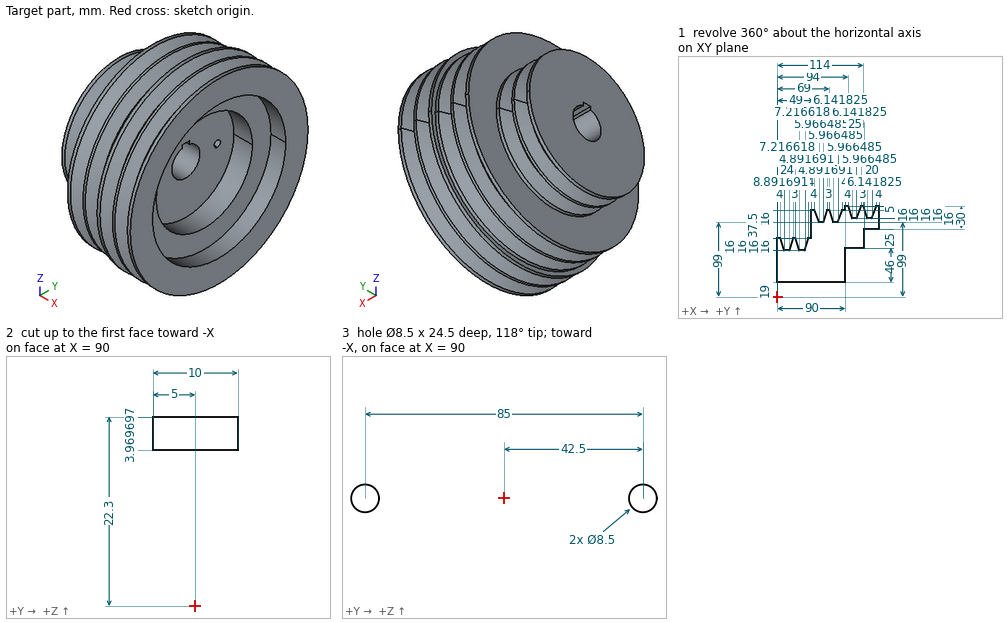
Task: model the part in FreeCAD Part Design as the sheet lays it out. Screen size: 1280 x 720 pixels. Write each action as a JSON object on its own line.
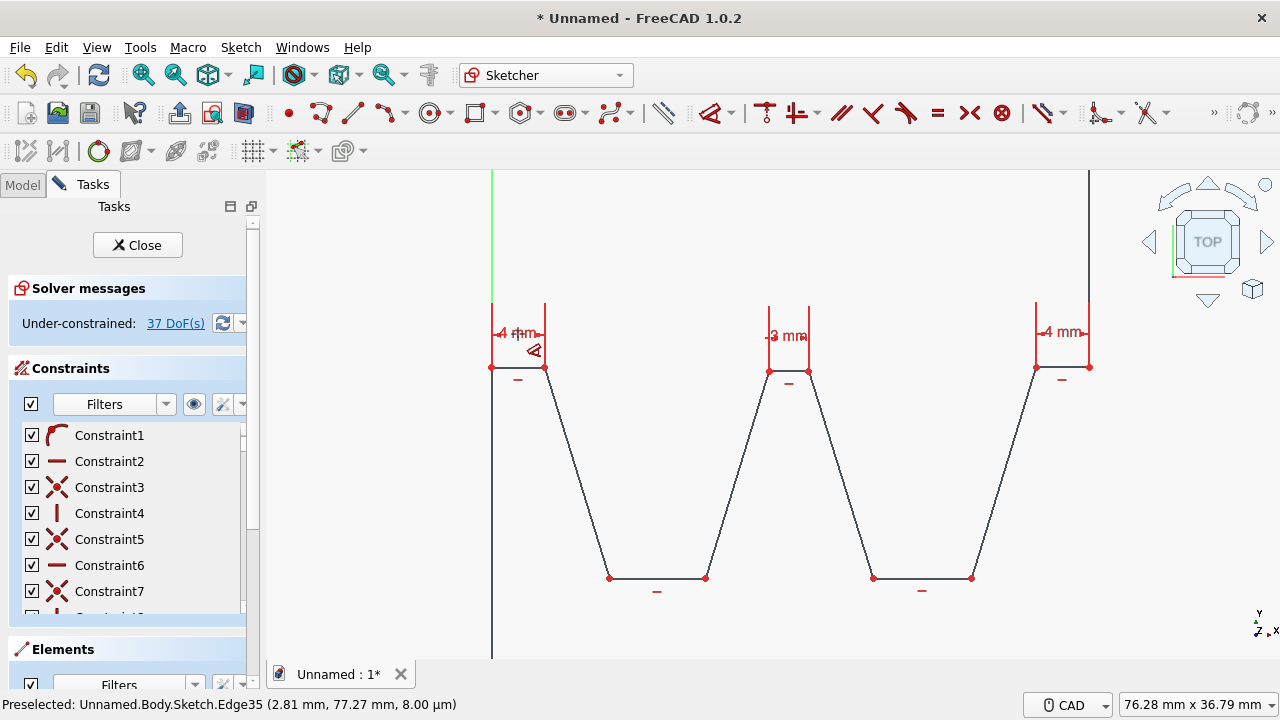
{"action": "scroll", "coordinate": [531, 368], "scroll_direction": "down", "scroll_amount": 8}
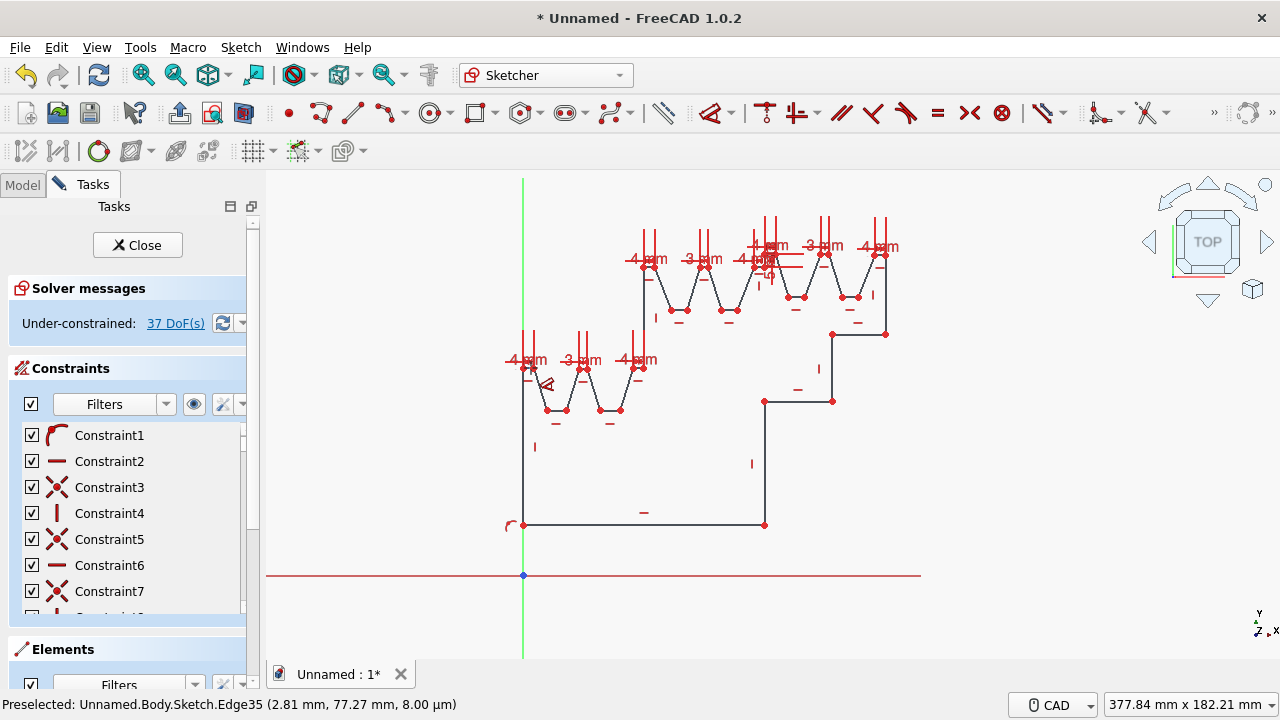
{"action": "left_click", "coordinate": [596, 525]}
{"action": "left_click", "coordinate": [644, 559]}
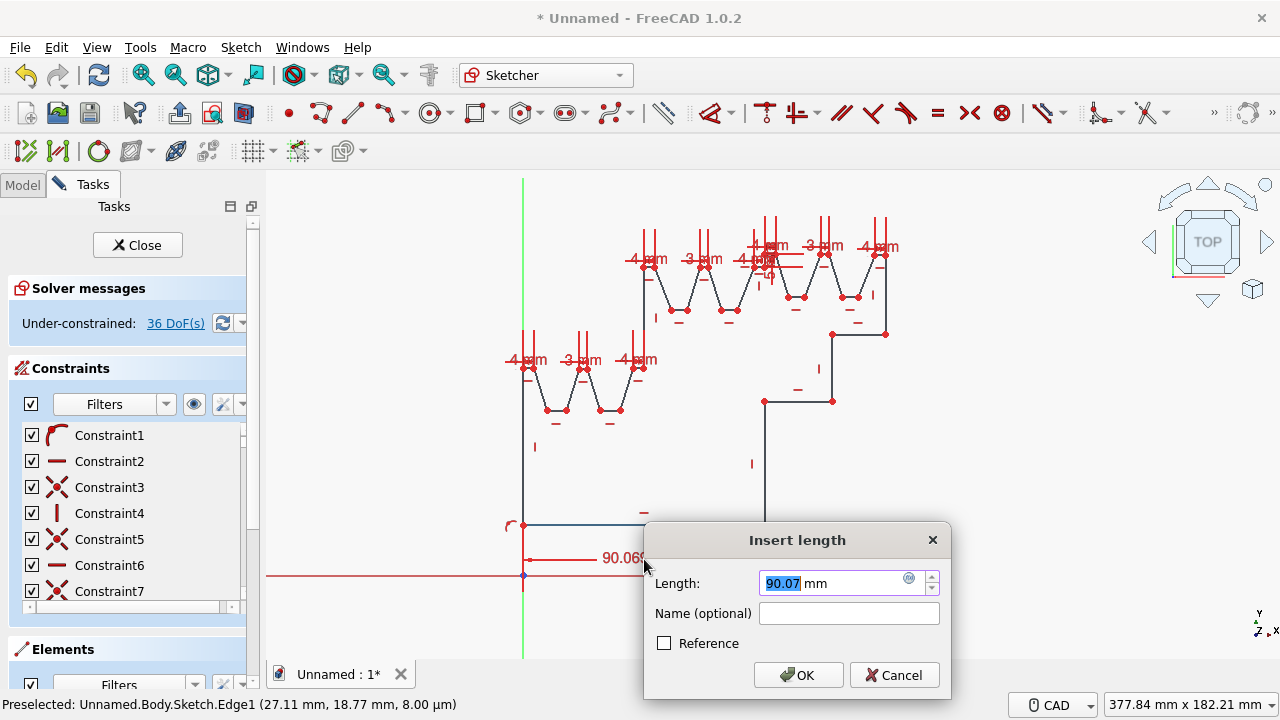
{"action": "type", "text": "90"}
{"action": "key", "text": "Return"}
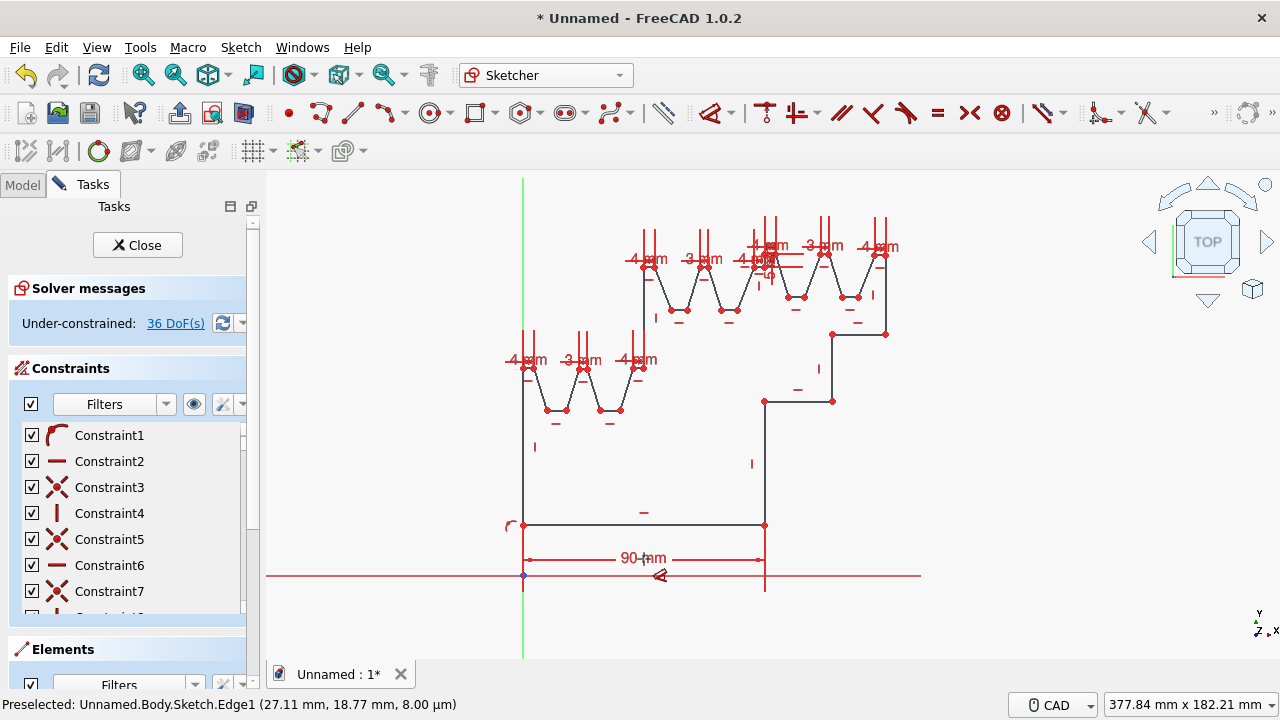
{"action": "left_click", "coordinate": [765, 488]}
{"action": "left_click", "coordinate": [799, 464]}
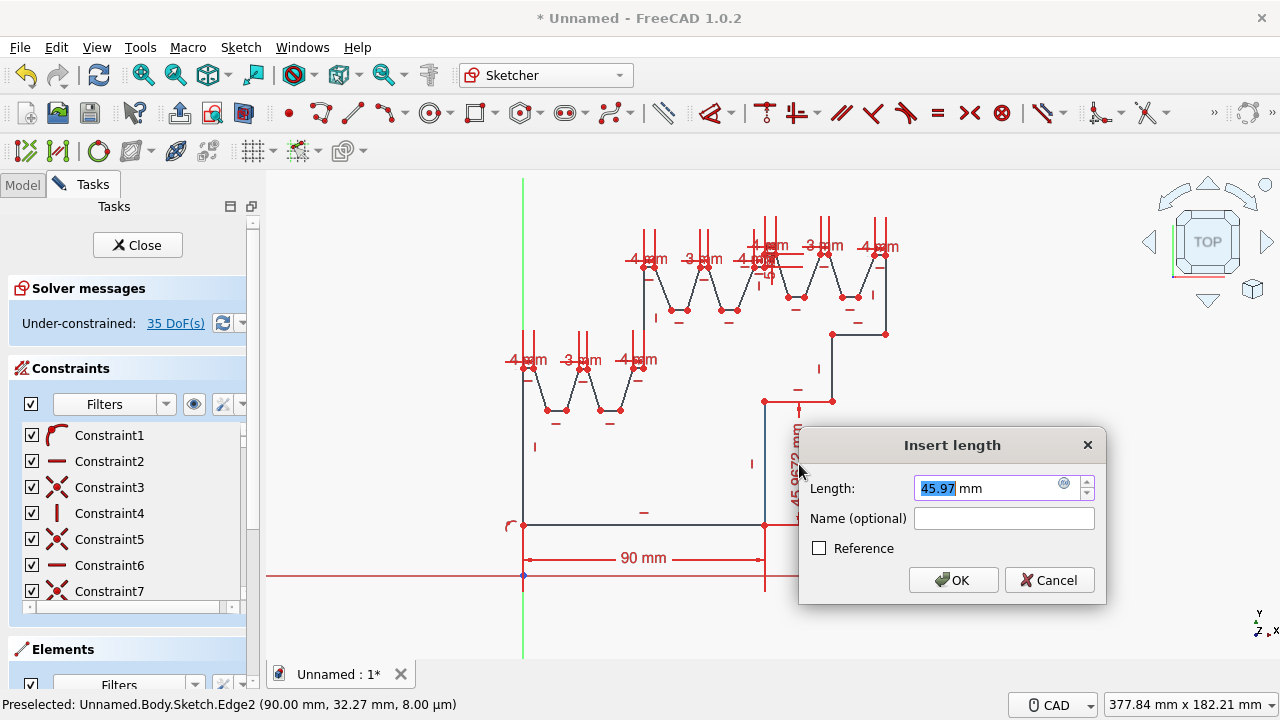
{"action": "type", "text": "46"}
{"action": "key", "text": "Return"}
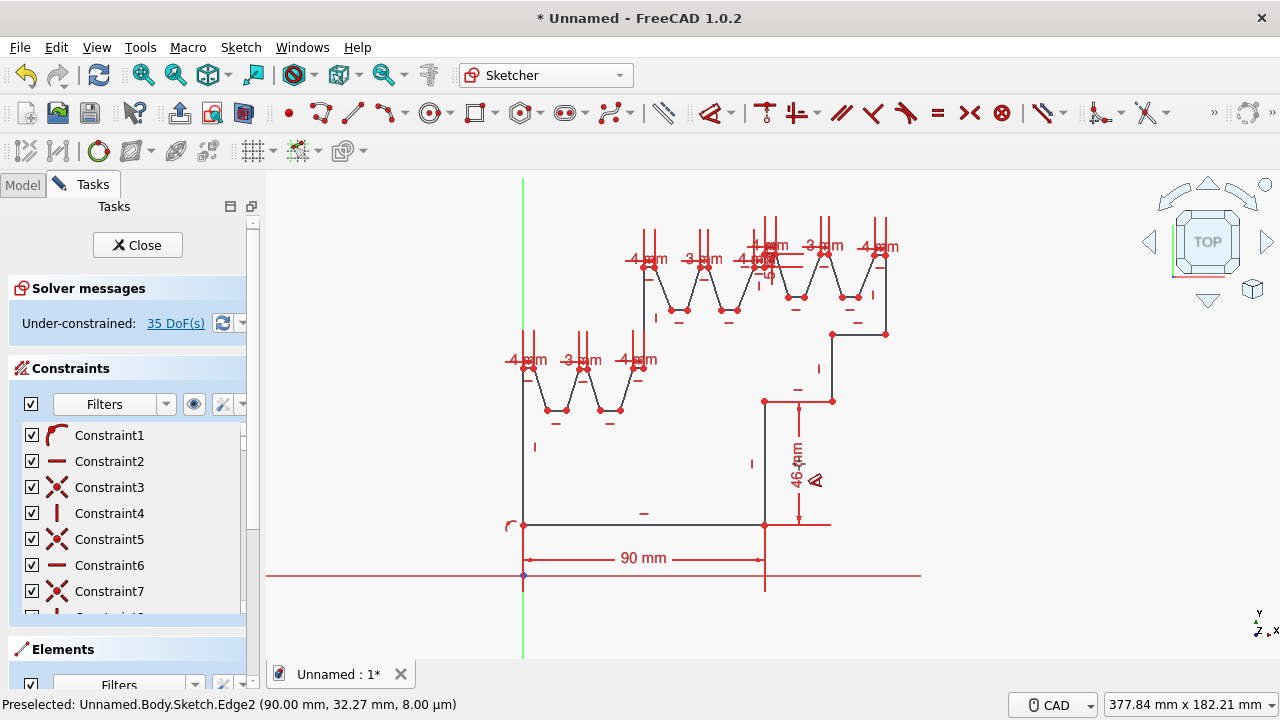
{"action": "left_click", "coordinate": [785, 402]}
{"action": "left_click", "coordinate": [798, 368]}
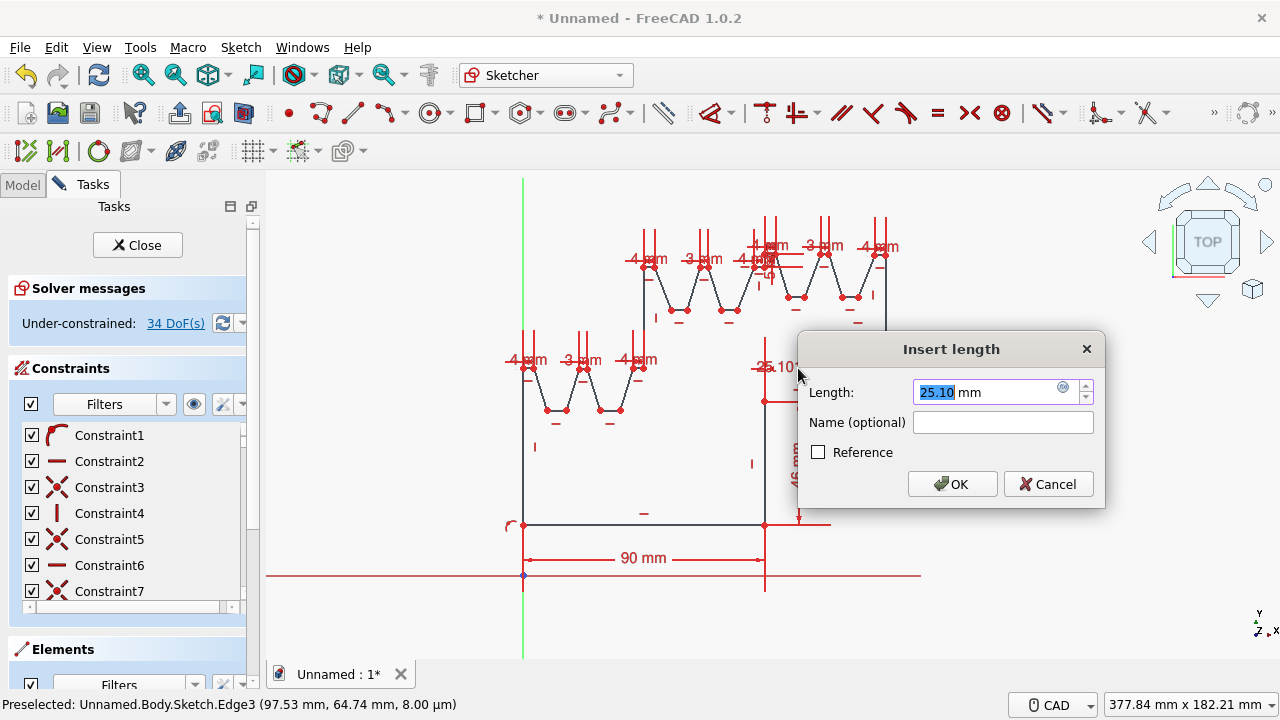
{"action": "type", "text": "25"}
{"action": "key", "text": "Return"}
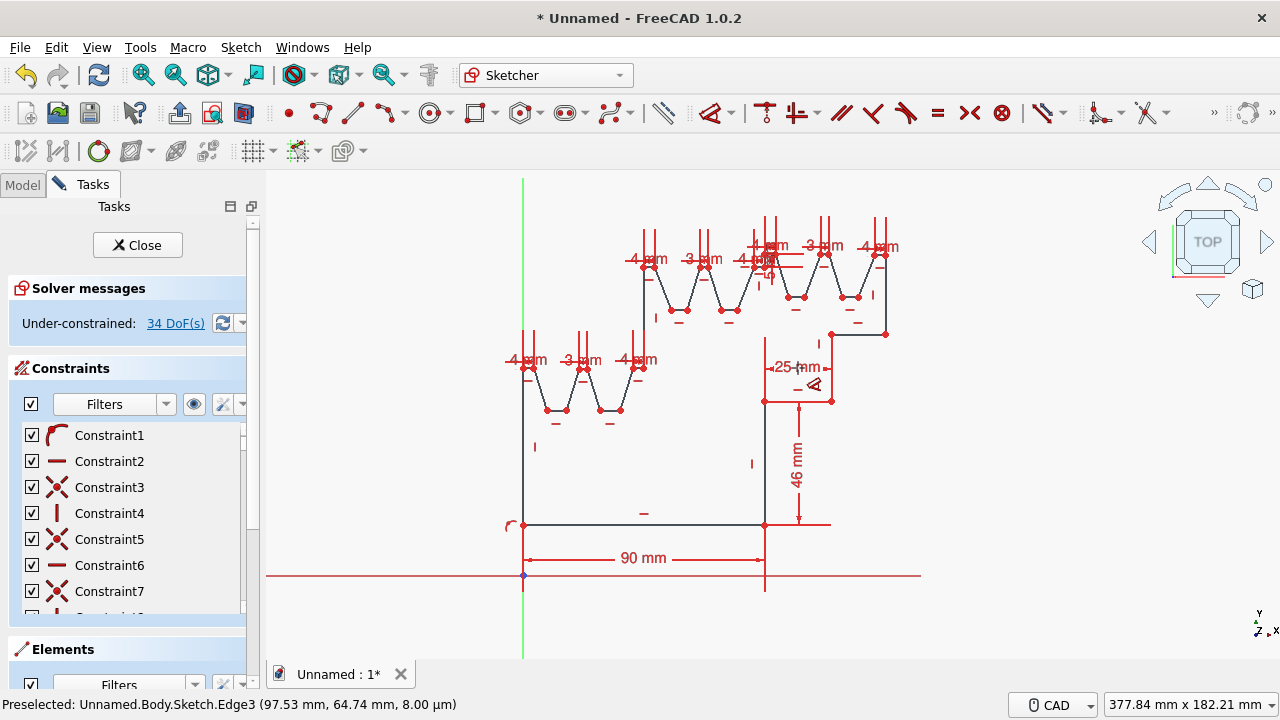
{"action": "left_click", "coordinate": [832, 382]}
{"action": "left_click", "coordinate": [866, 392]}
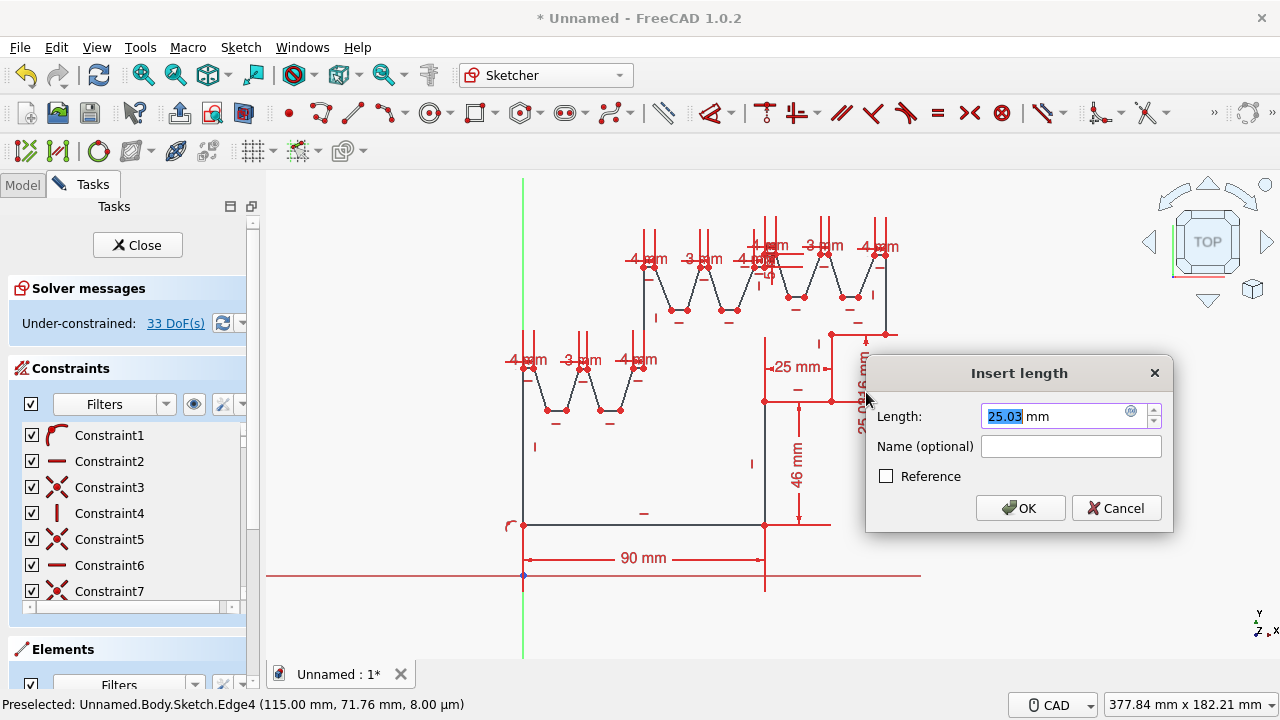
{"action": "type", "text": "25"}
{"action": "key", "text": "Return"}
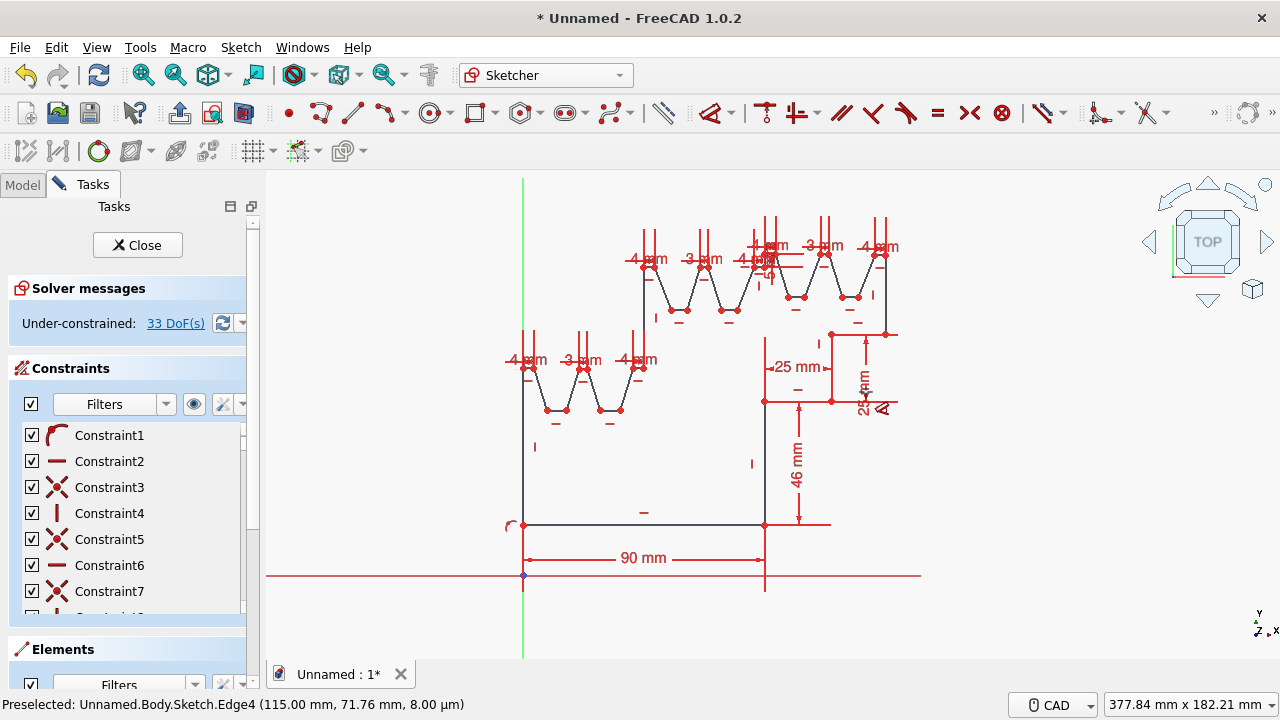
{"action": "left_click", "coordinate": [848, 335]}
{"action": "left_click", "coordinate": [871, 301]}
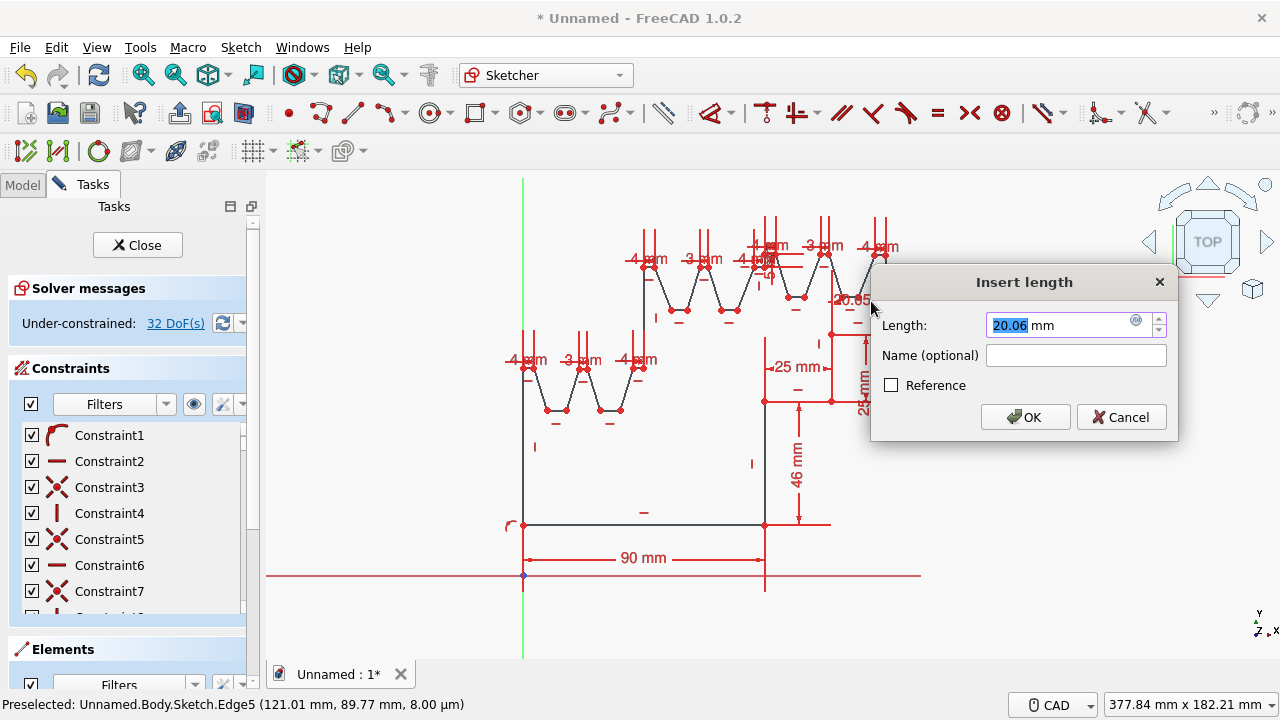
{"action": "type", "text": "20"}
{"action": "key", "text": "Return"}